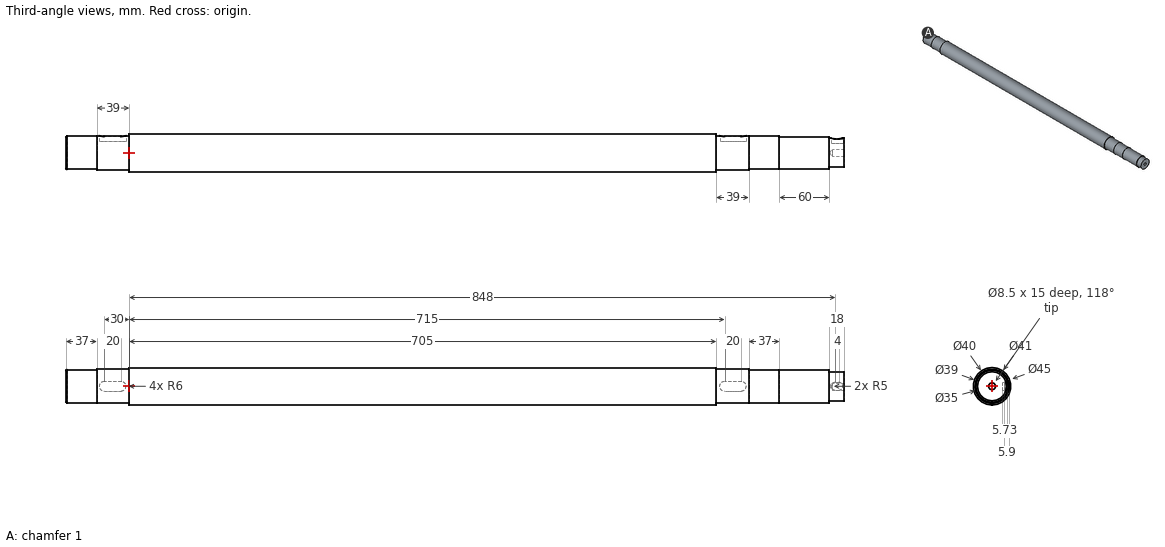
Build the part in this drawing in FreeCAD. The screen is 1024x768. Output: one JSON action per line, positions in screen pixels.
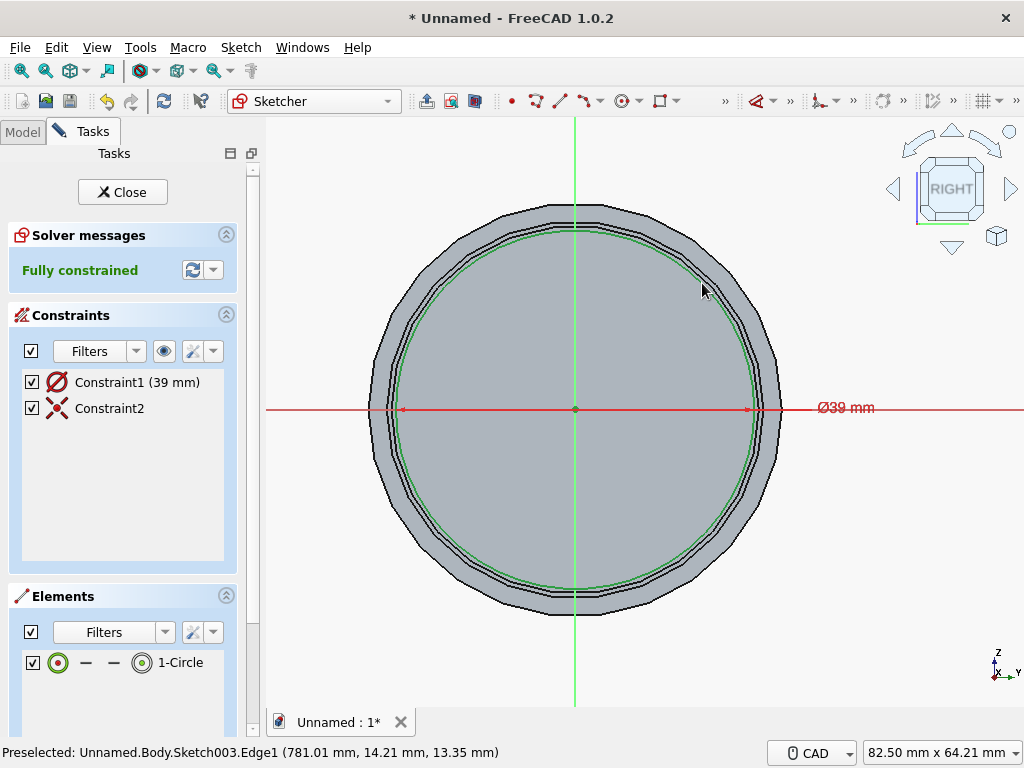
{"action": "left_click", "coordinate": [123, 192]}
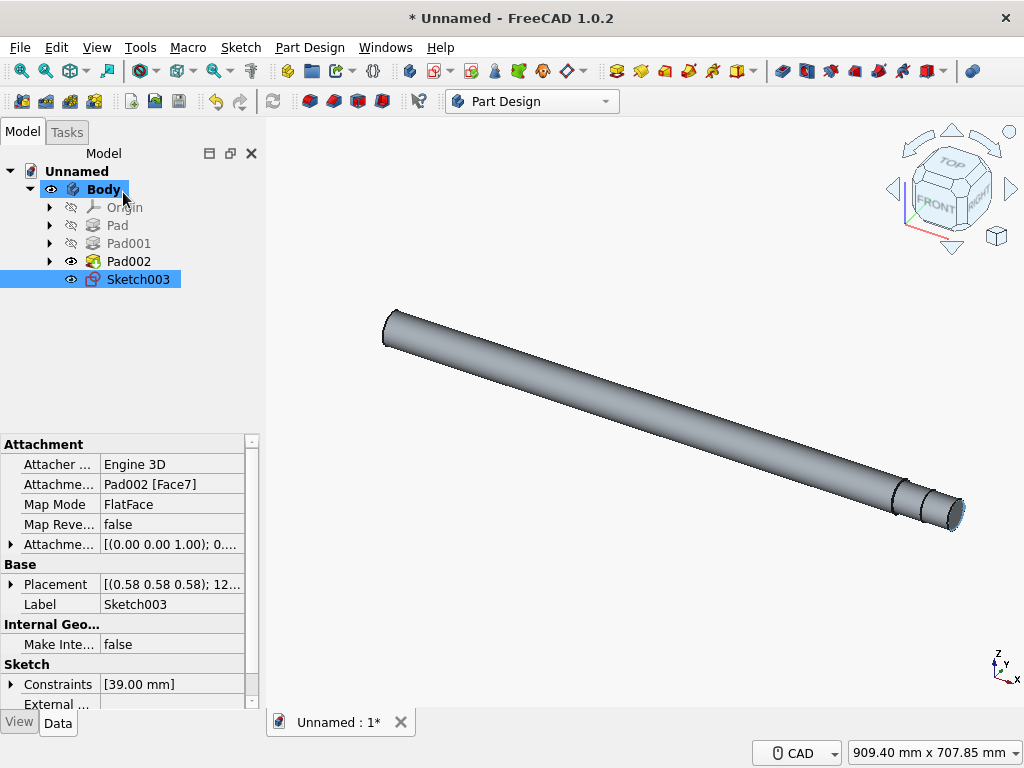
{"action": "left_click", "coordinate": [618, 72]}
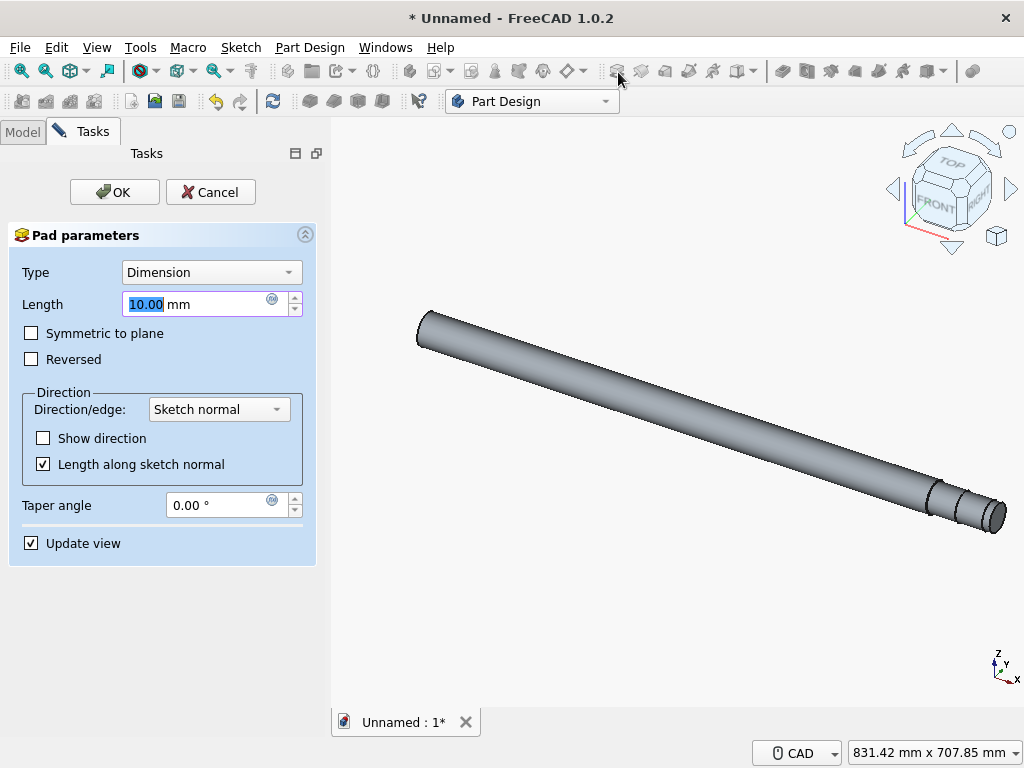
{"action": "type", "text": "60"}
{"action": "key", "text": "Tab"}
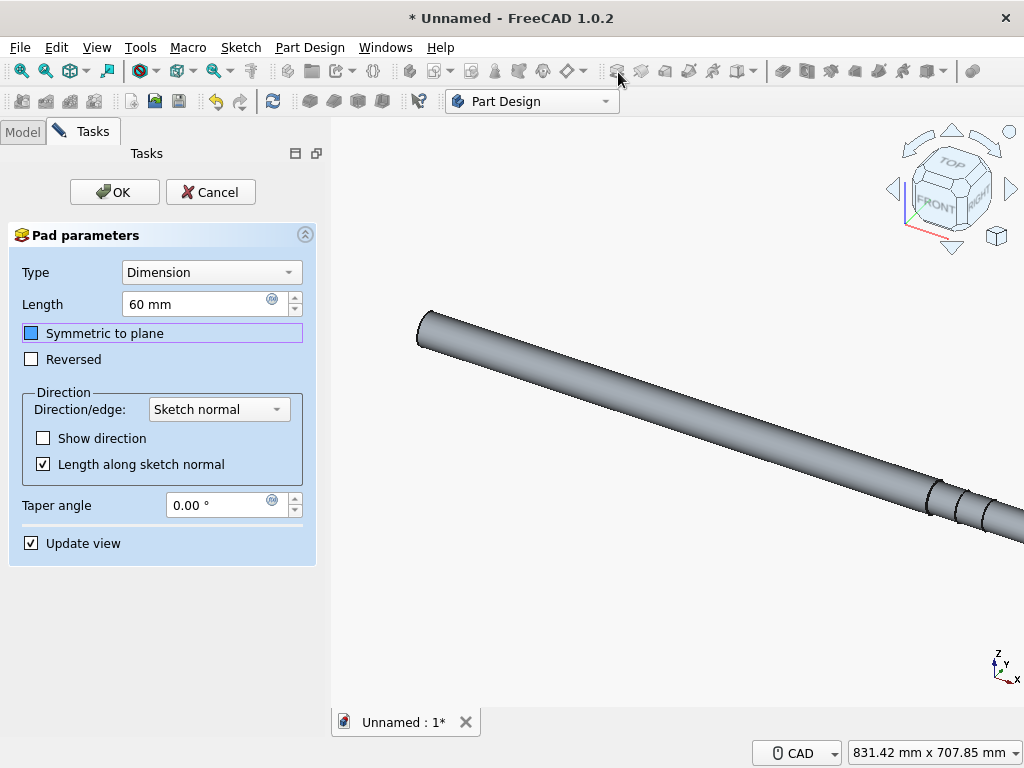
{"action": "left_click", "coordinate": [115, 192]}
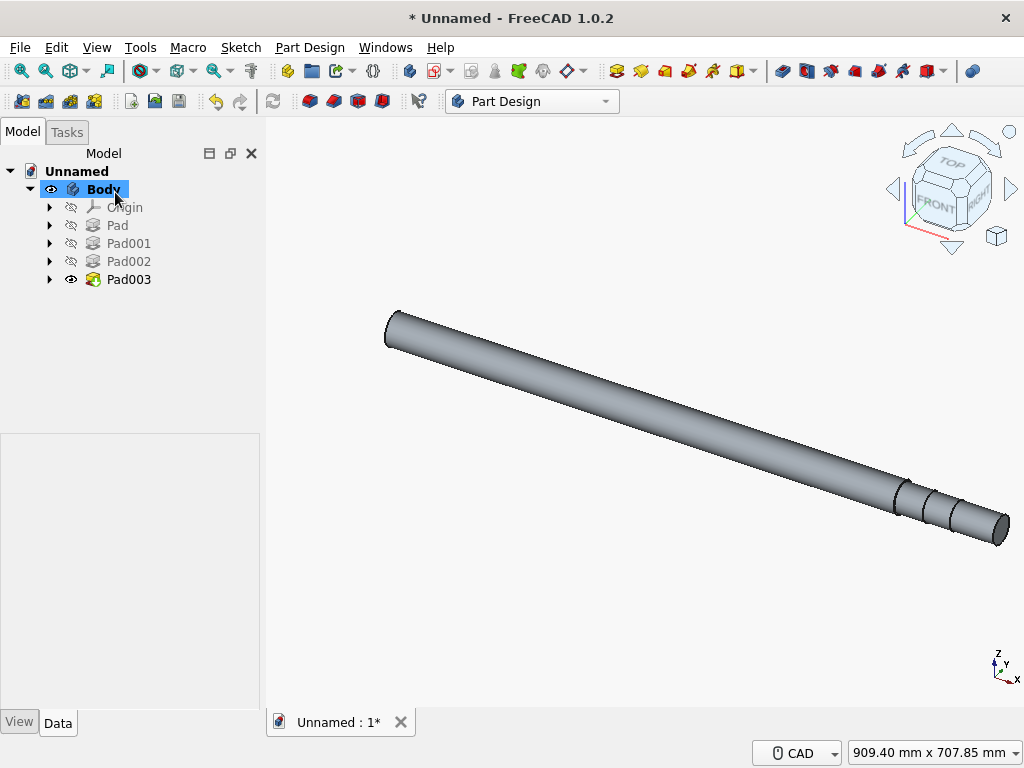
{"action": "key", "text": "0"}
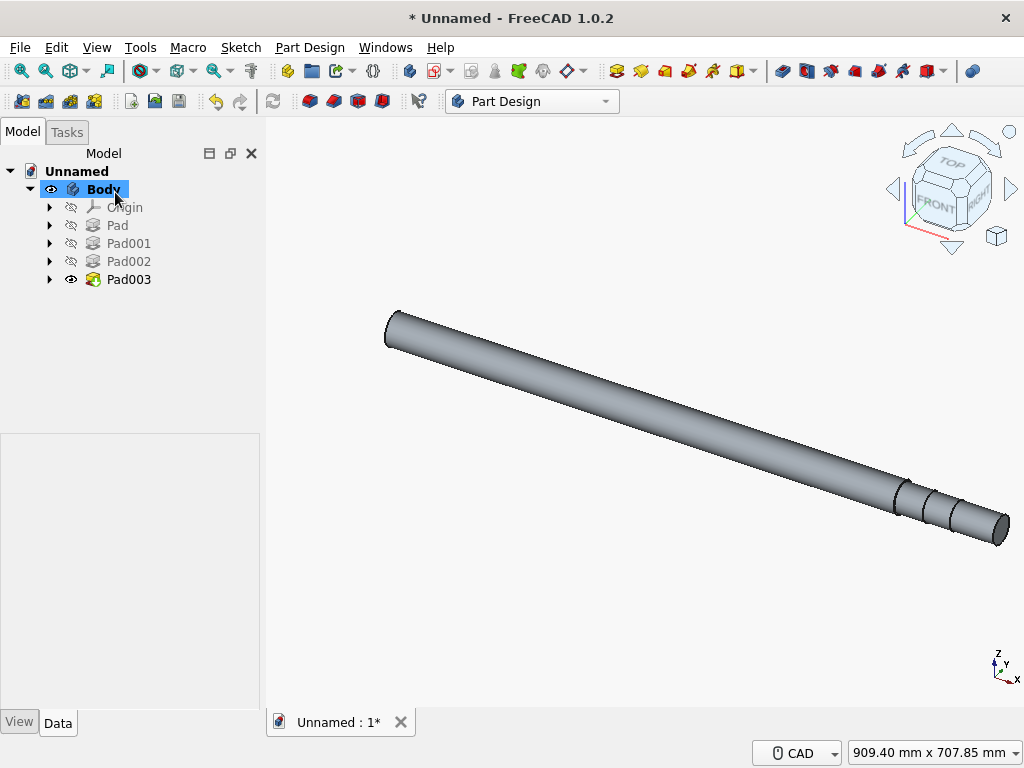
{"action": "left_click", "coordinate": [939, 579]}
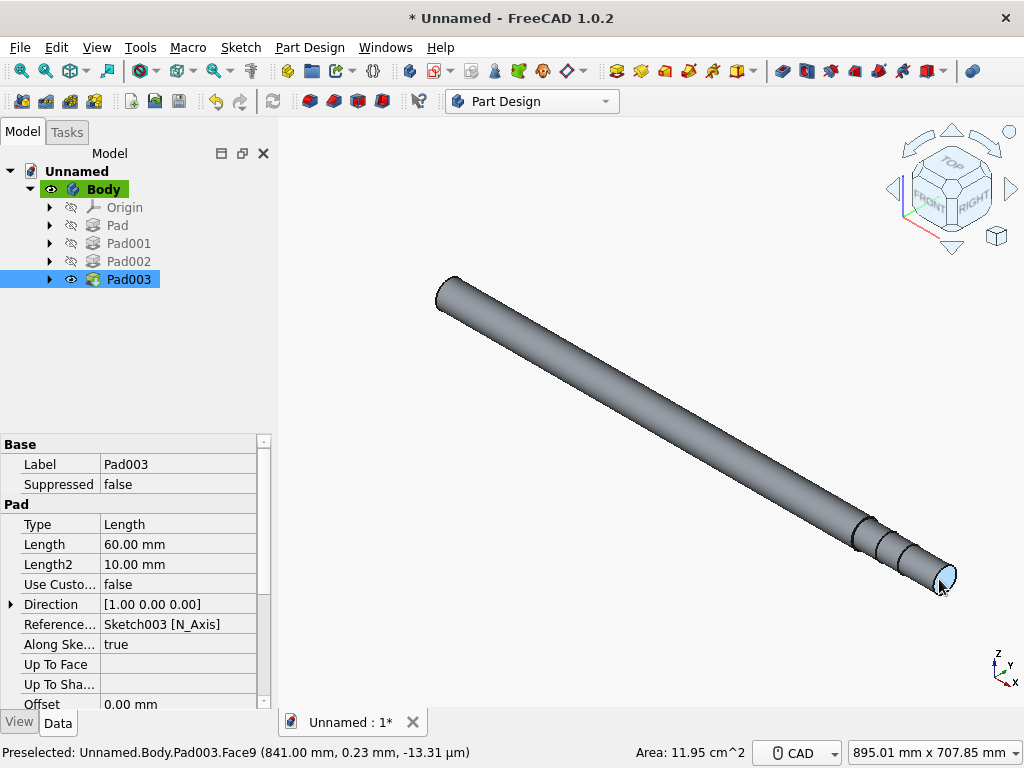
{"action": "left_click", "coordinate": [434, 72]}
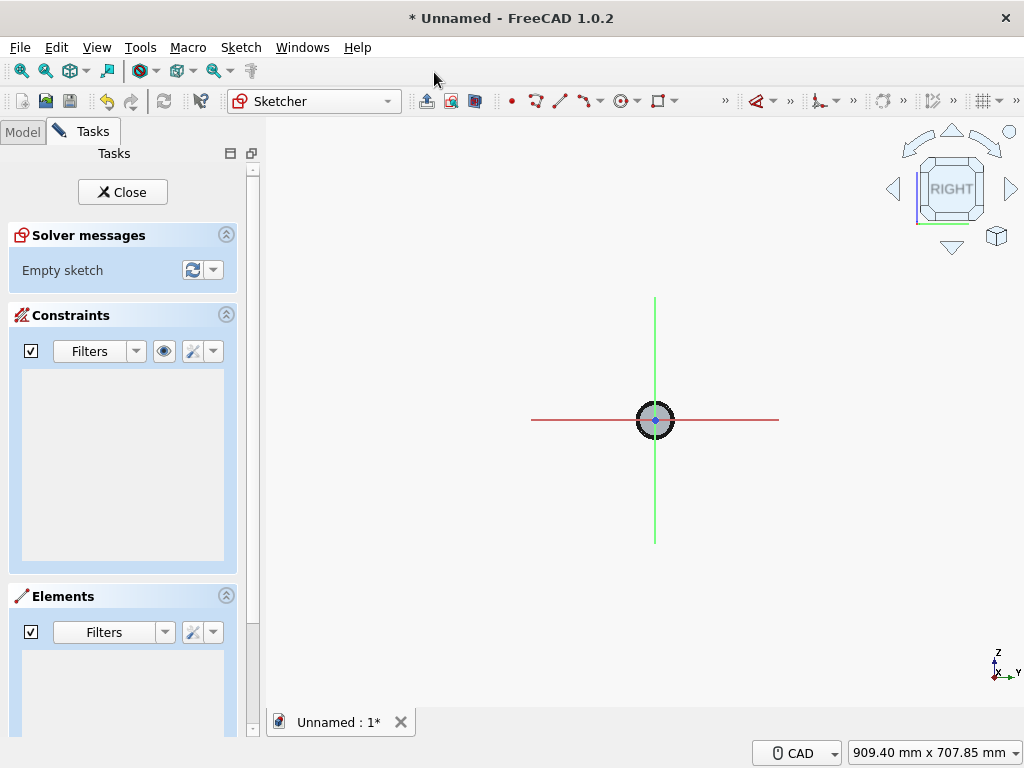
{"action": "scroll", "coordinate": [661, 421], "scroll_direction": "up", "scroll_amount": 13}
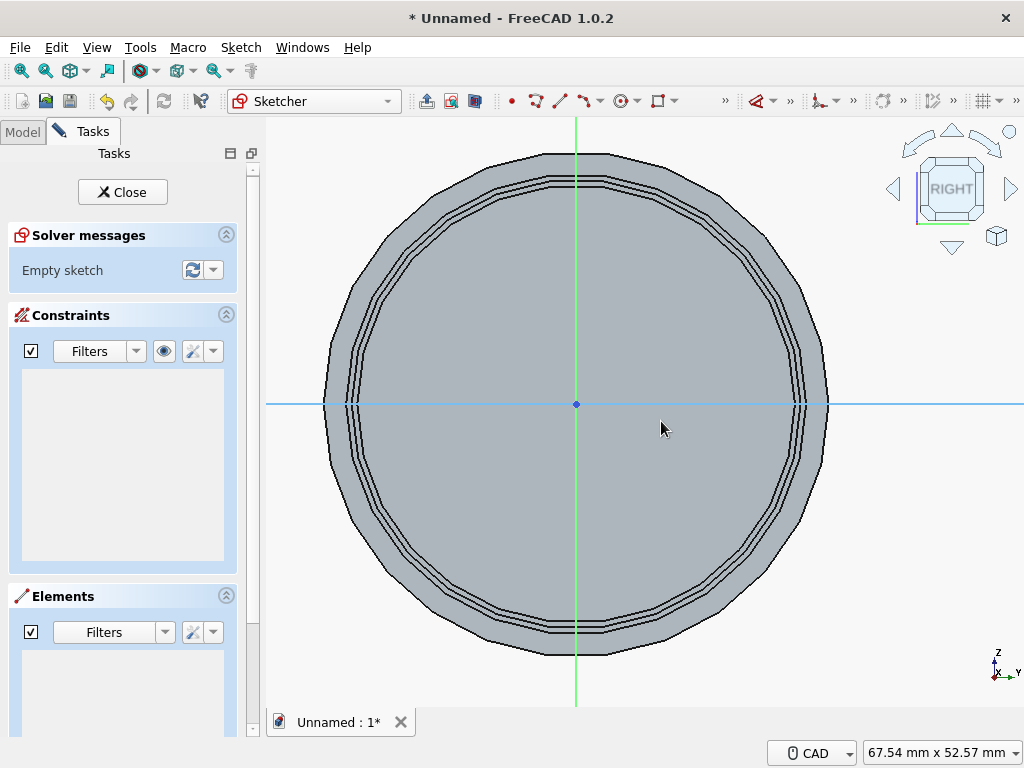
{"action": "left_click", "coordinate": [622, 102]}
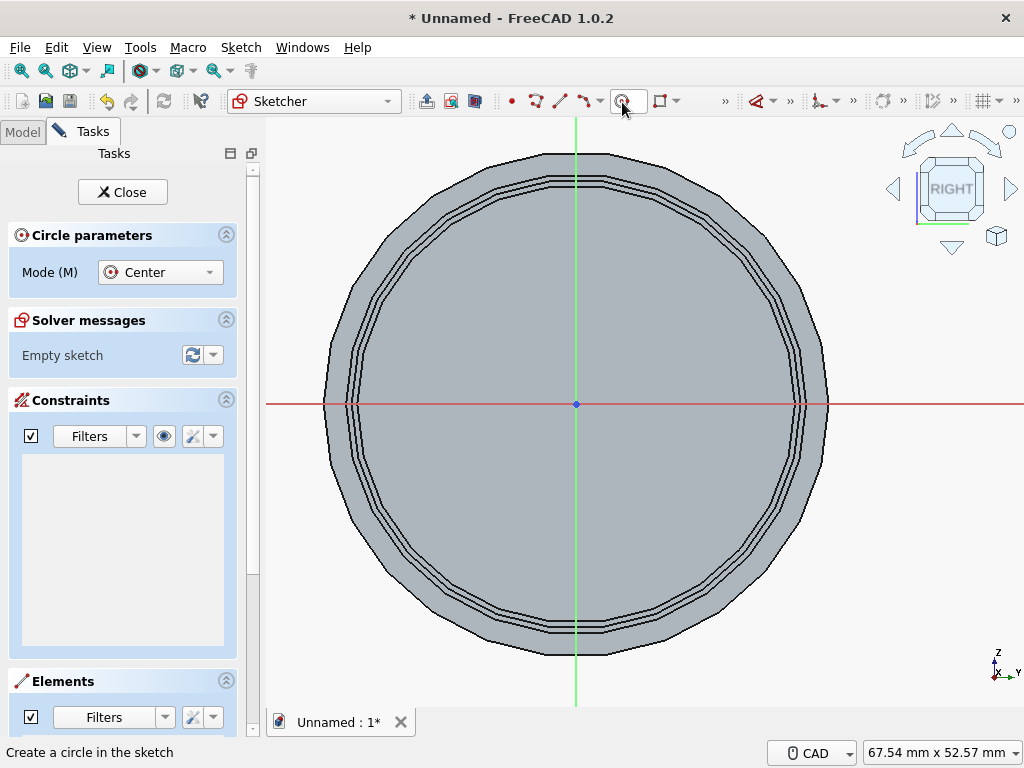
{"action": "left_click", "coordinate": [576, 404]}
{"action": "mouse_move", "coordinate": [715, 265]}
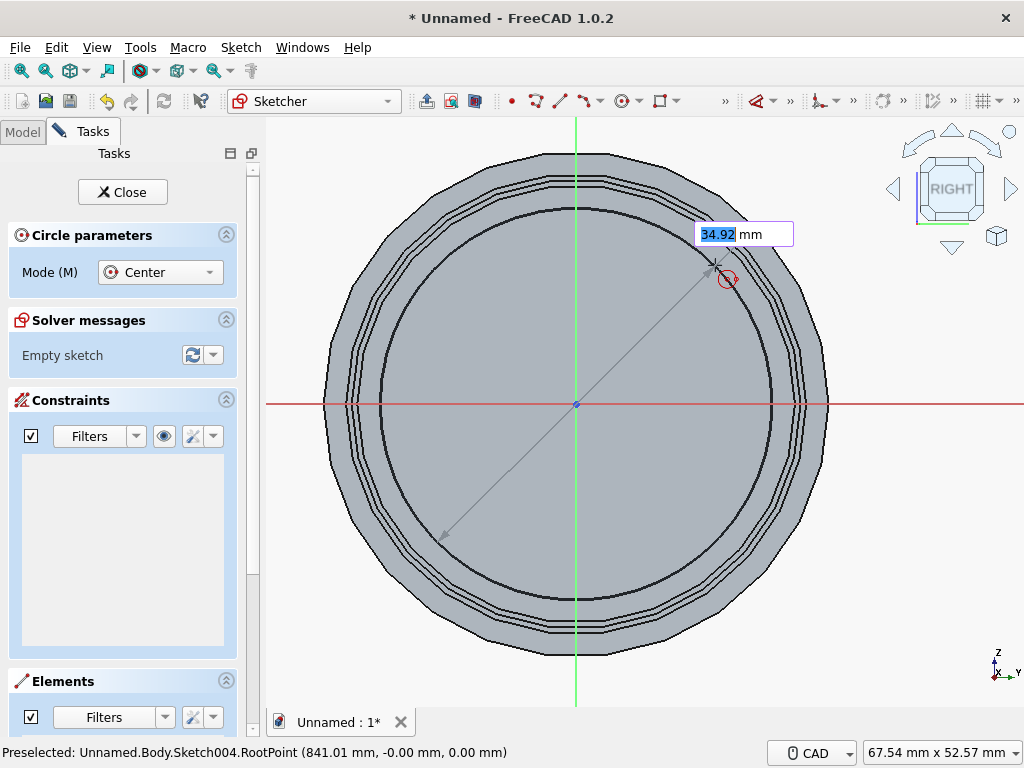
{"action": "type", "text": "35"}
{"action": "key", "text": "Return"}
{"action": "key", "text": "Escape"}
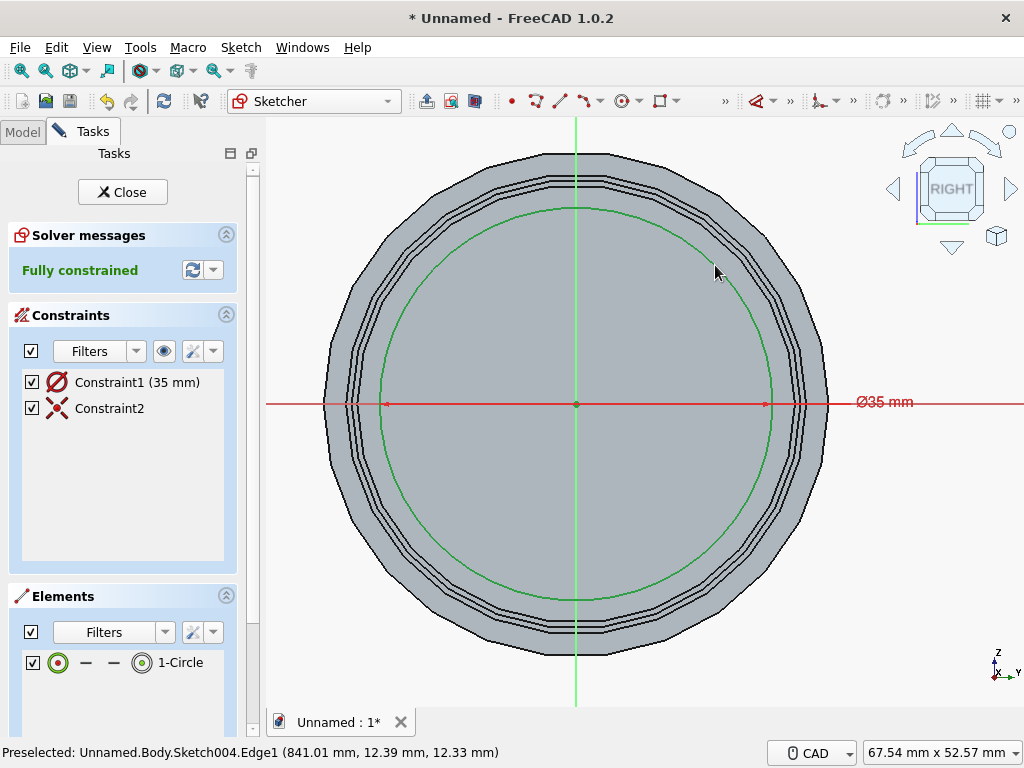
{"action": "left_click", "coordinate": [123, 192]}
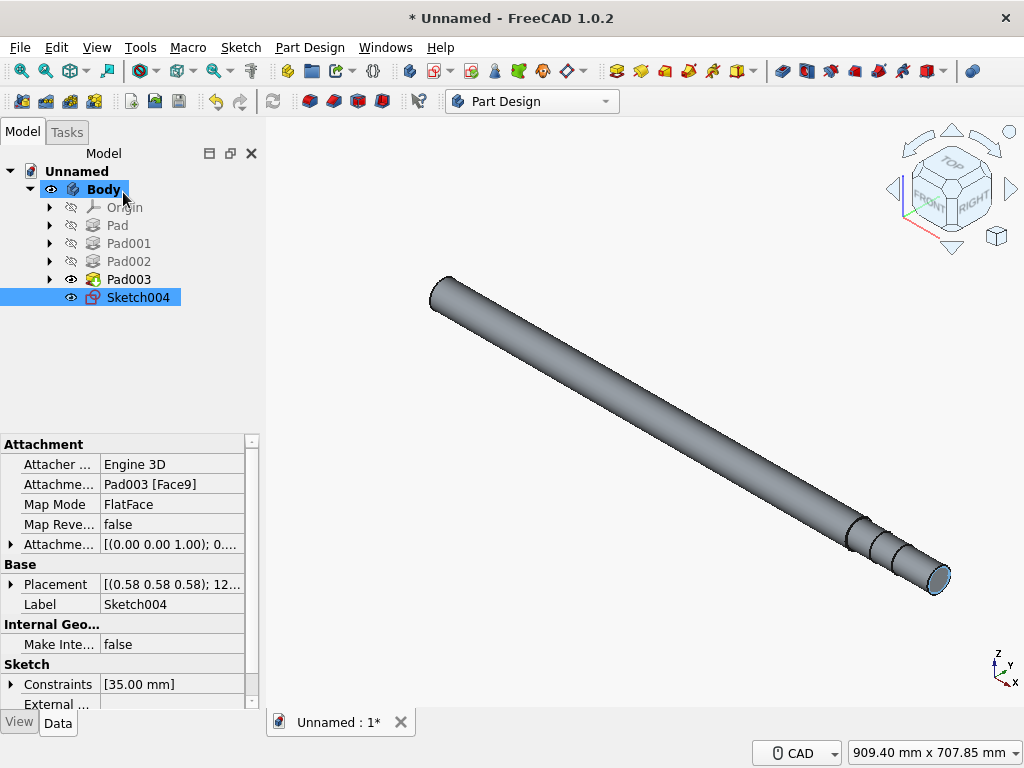
{"action": "left_click", "coordinate": [618, 72]}